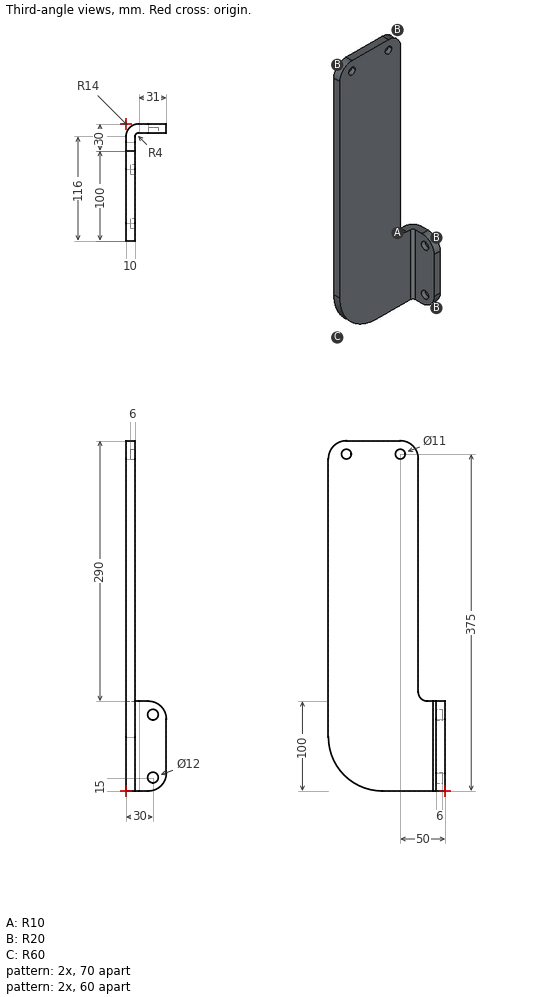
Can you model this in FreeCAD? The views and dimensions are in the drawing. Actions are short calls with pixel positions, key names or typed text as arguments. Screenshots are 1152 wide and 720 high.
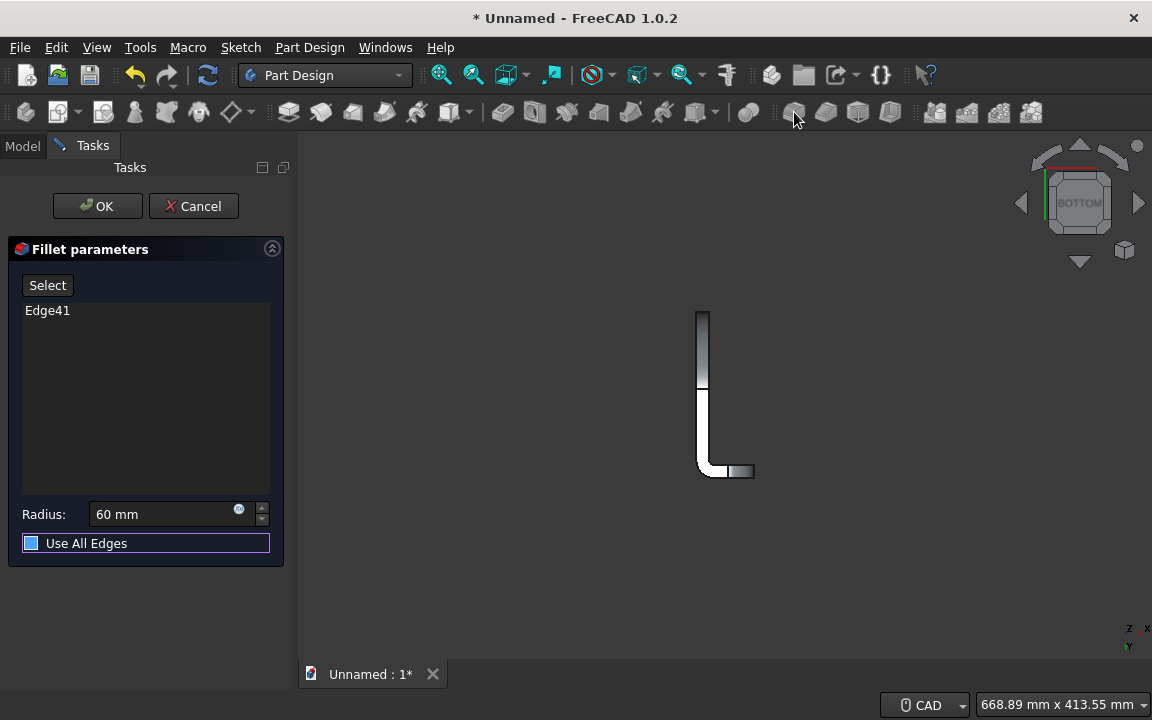
click(98, 206)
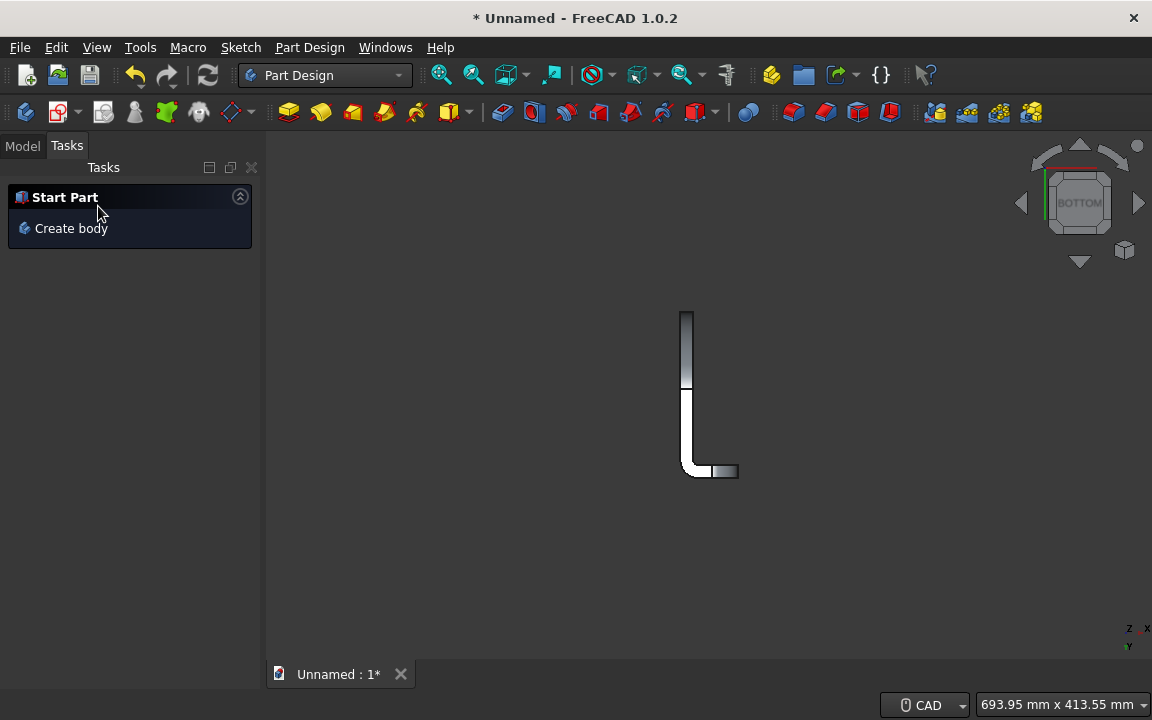
click(442, 76)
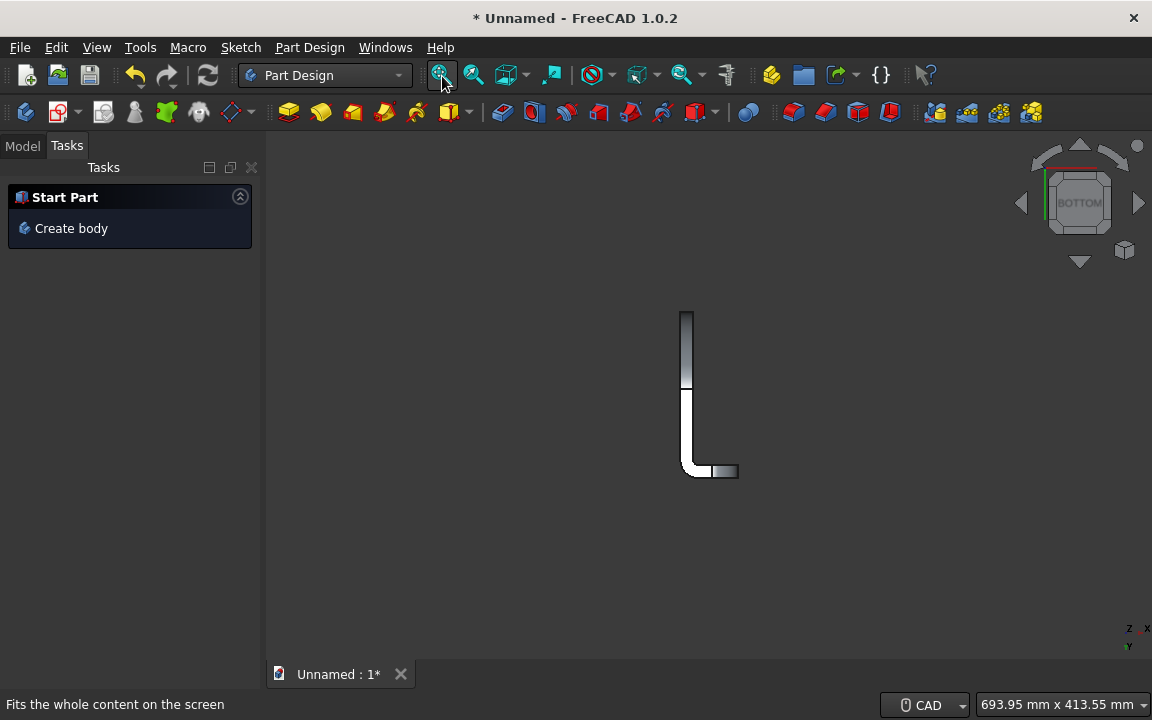
key(0)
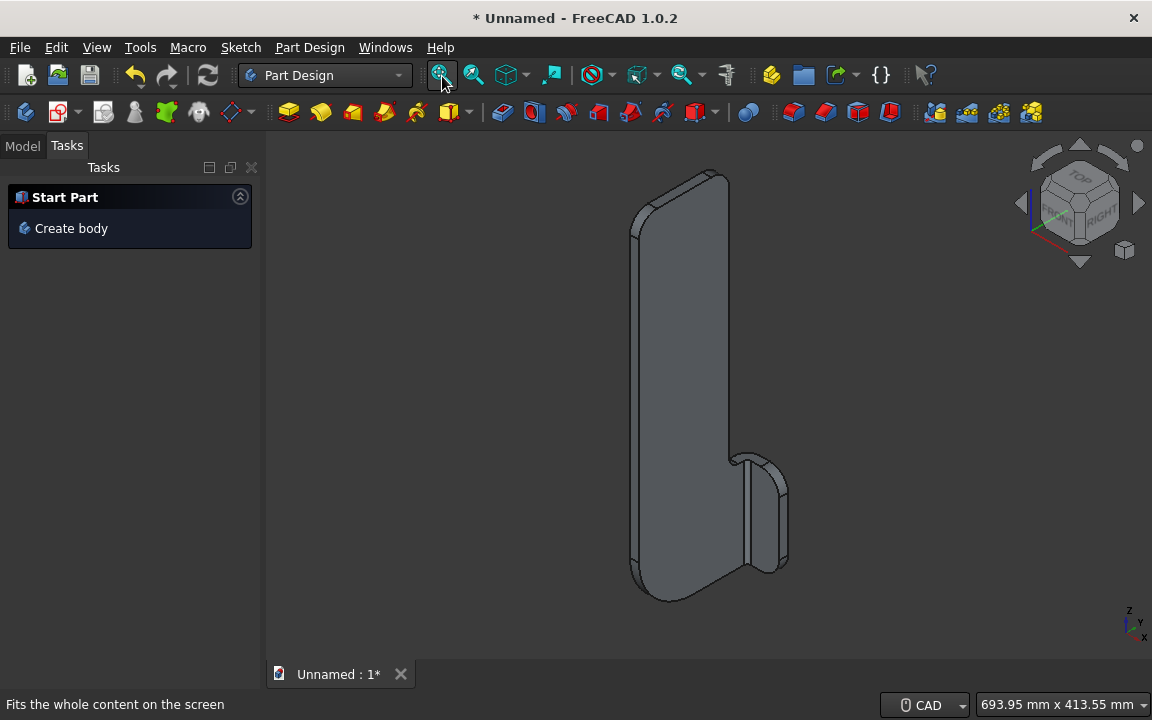
click(765, 490)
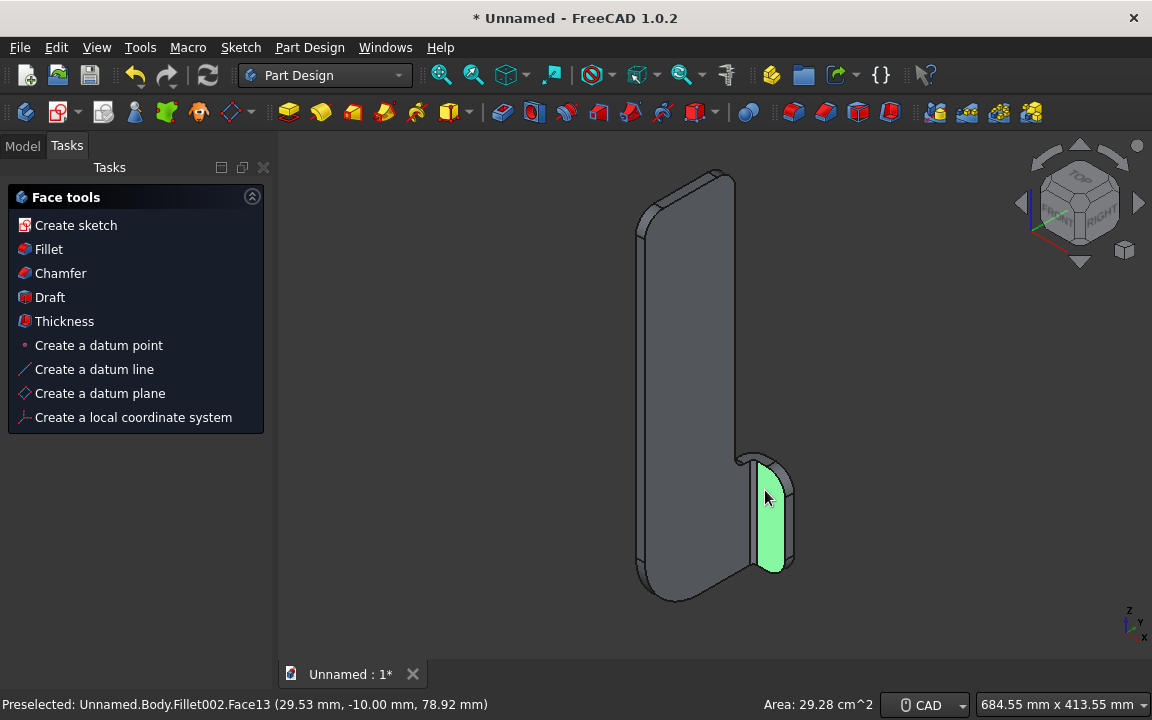
click(58, 112)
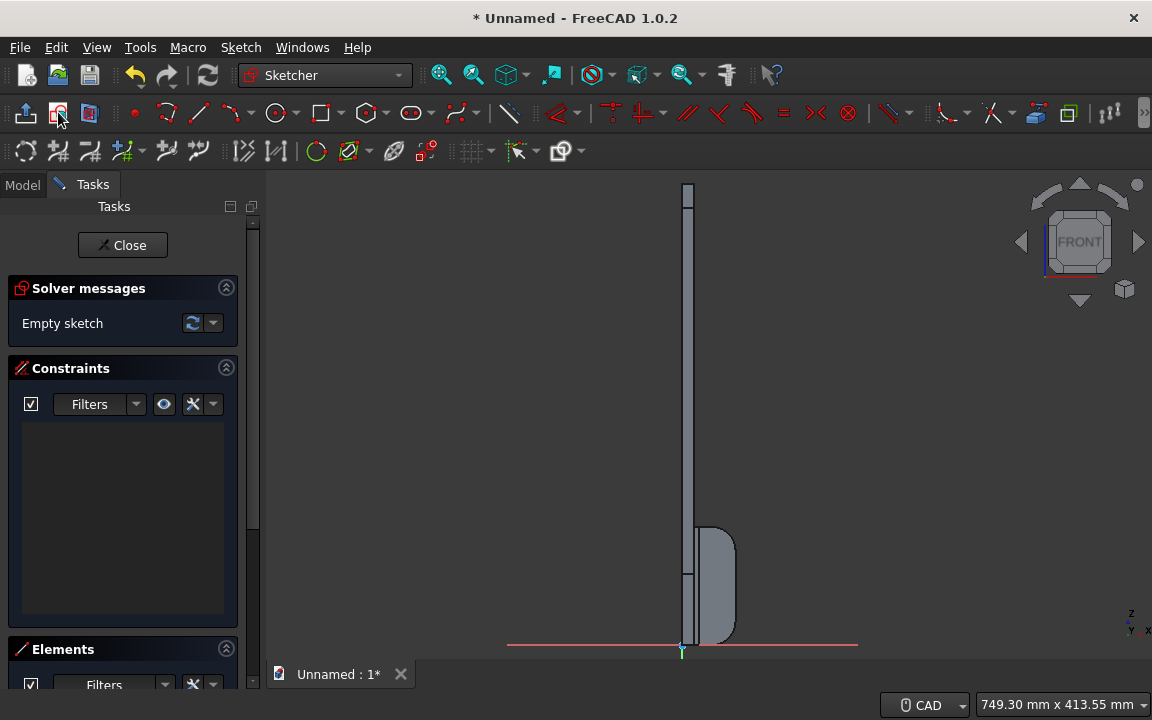
click(90, 114)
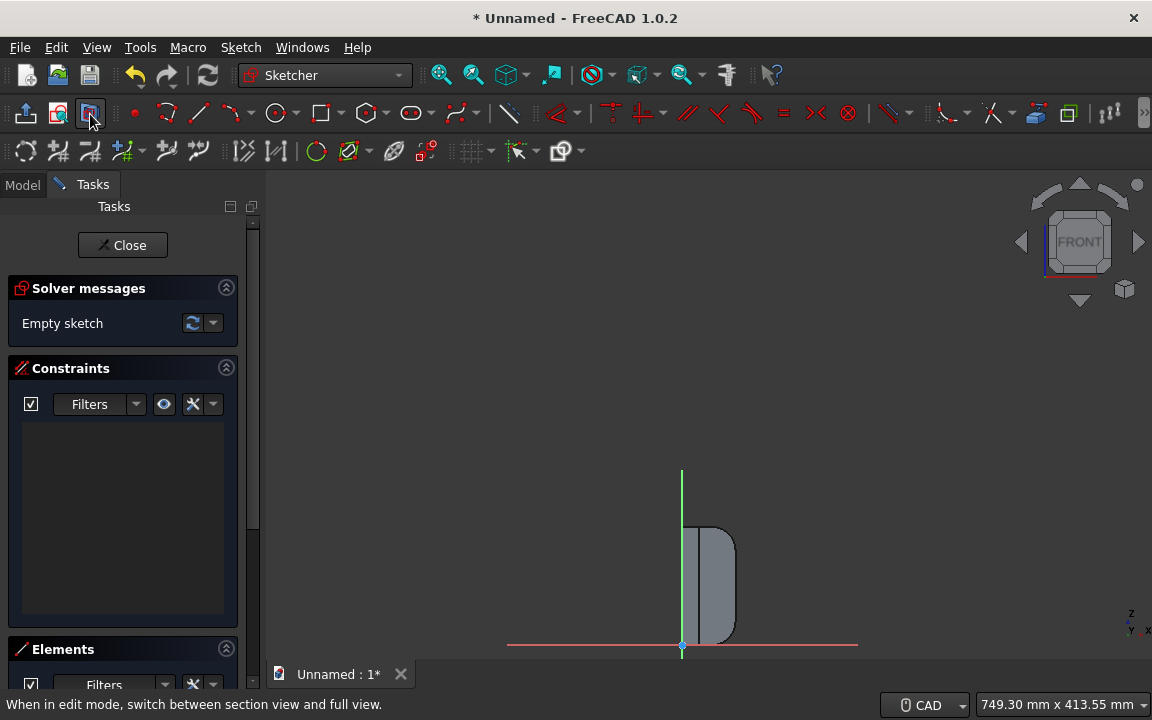
scroll(640, 414, down, 5)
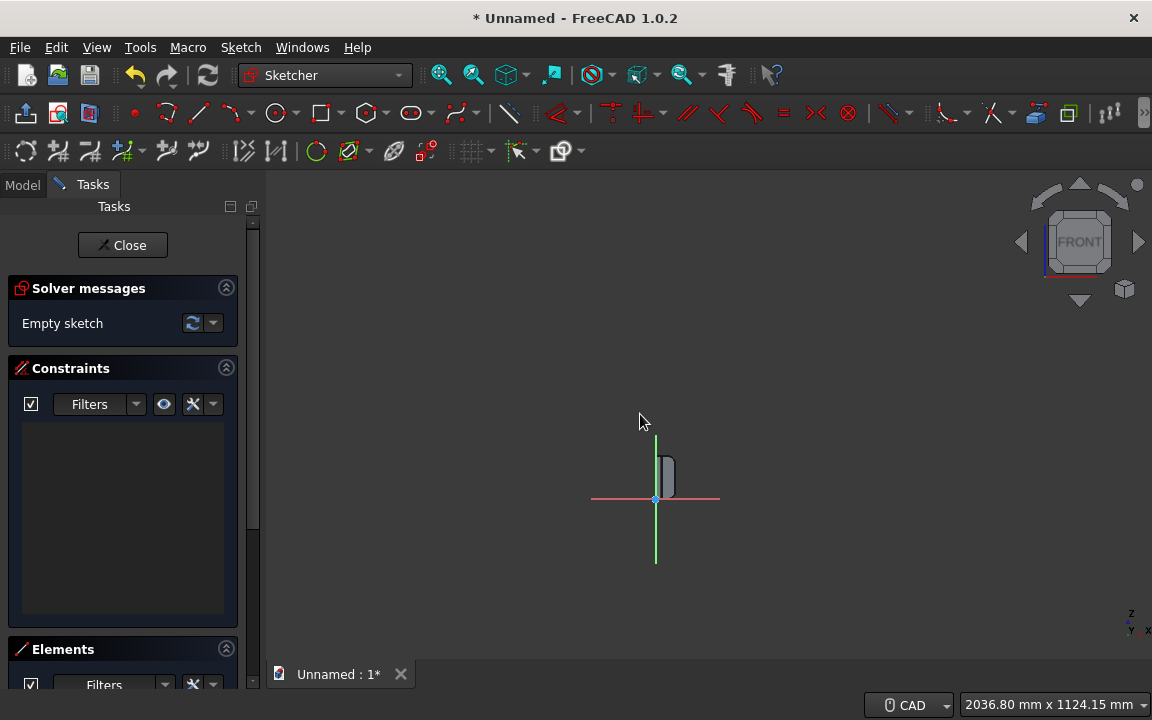
scroll(670, 497, up, 15)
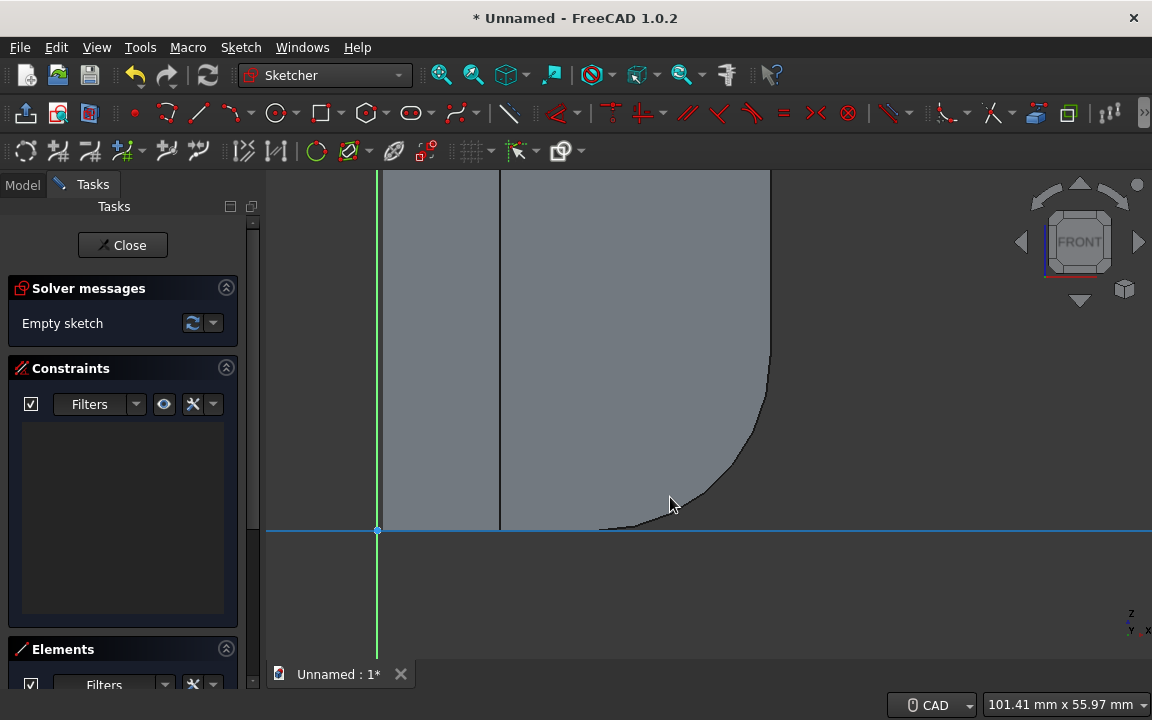
scroll(639, 391, up, 5)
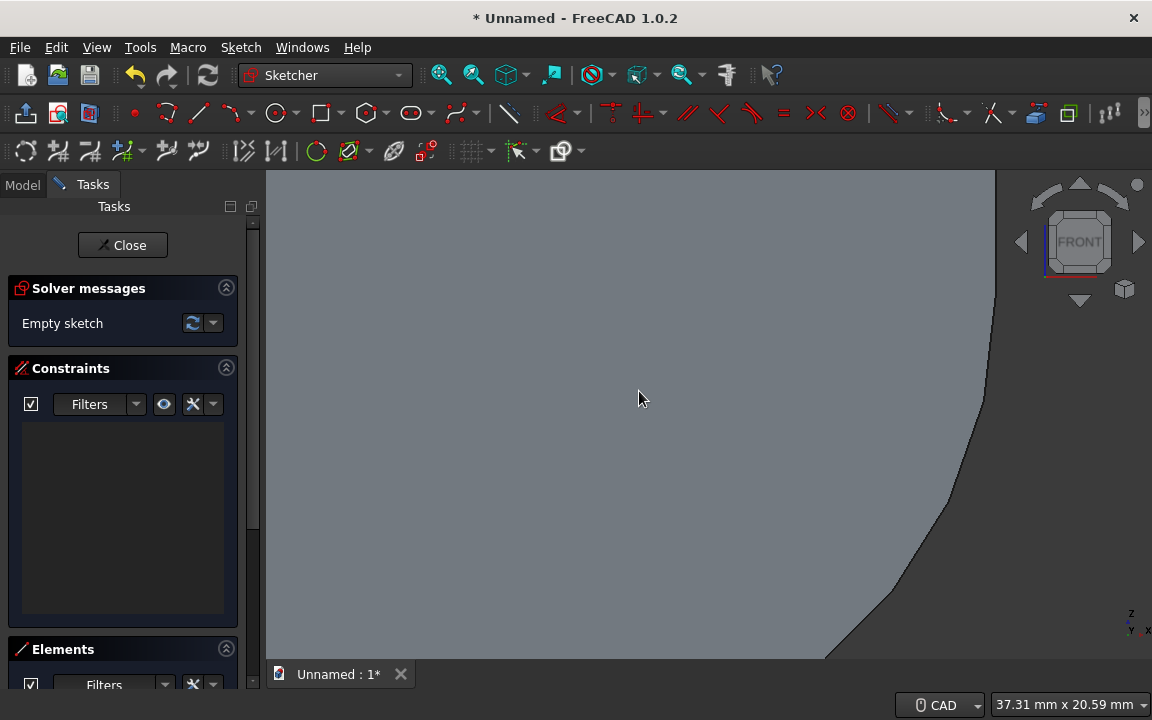
click(276, 114)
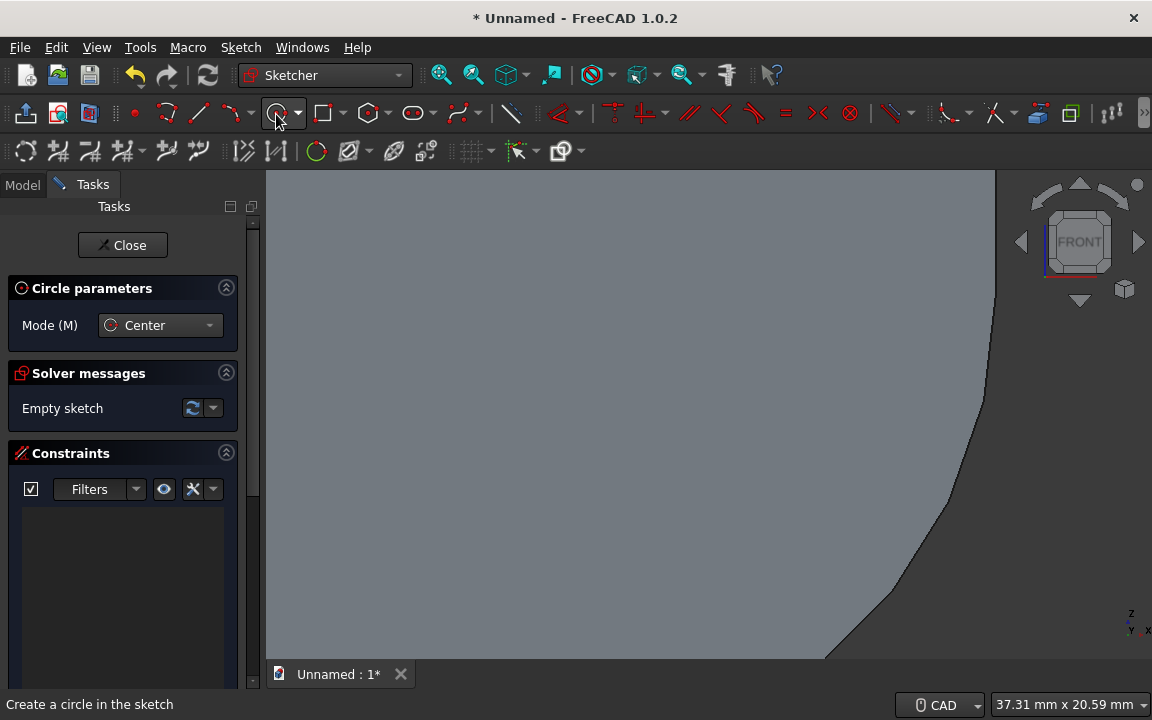
click(640, 414)
move(740, 313)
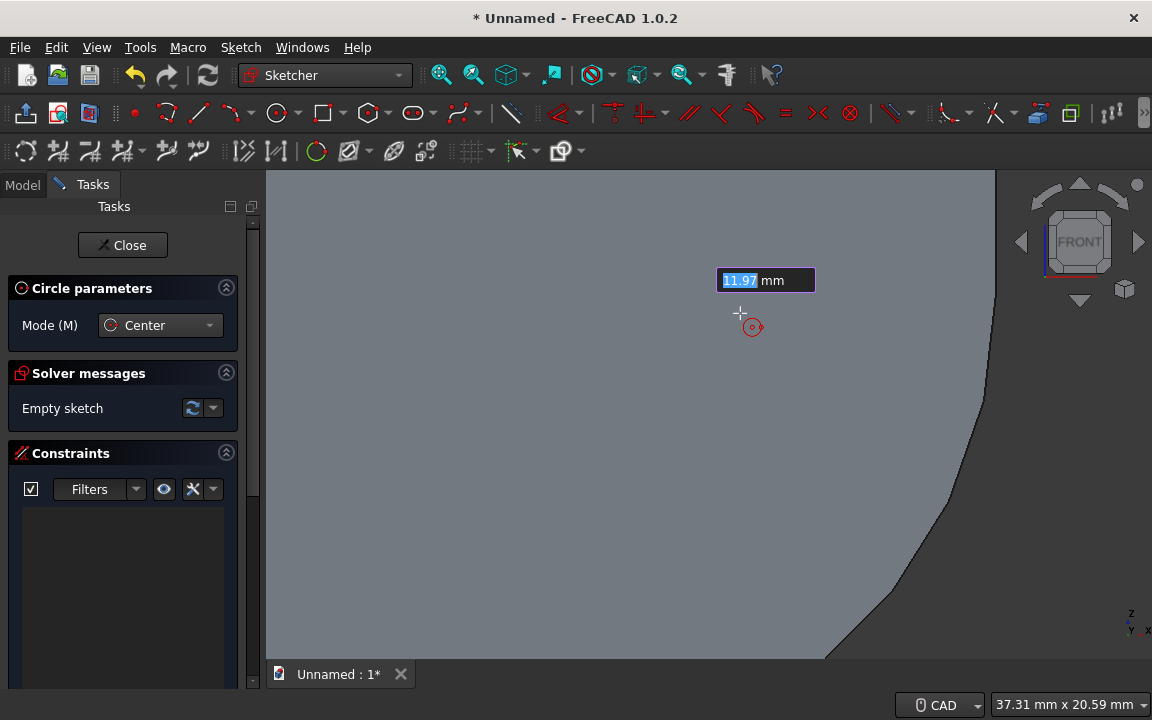
text(12)
key(Return)
key(Escape)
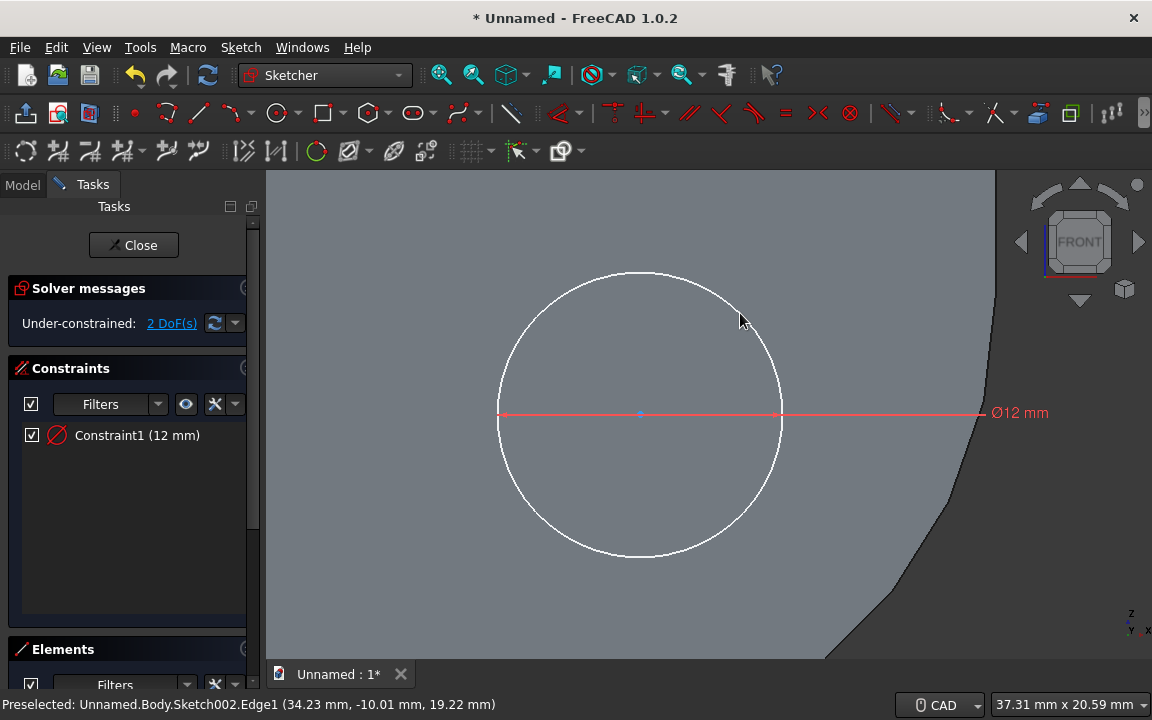
key(d)